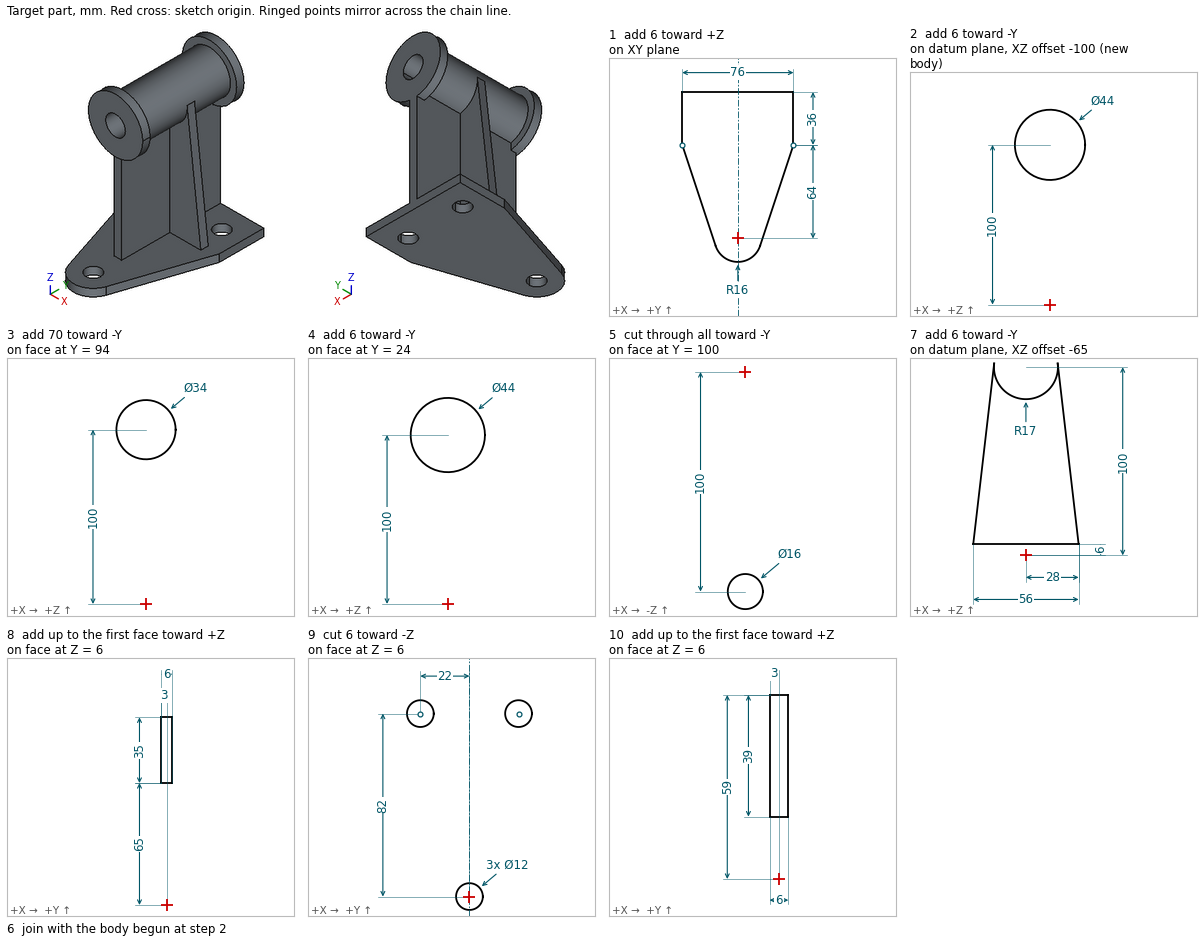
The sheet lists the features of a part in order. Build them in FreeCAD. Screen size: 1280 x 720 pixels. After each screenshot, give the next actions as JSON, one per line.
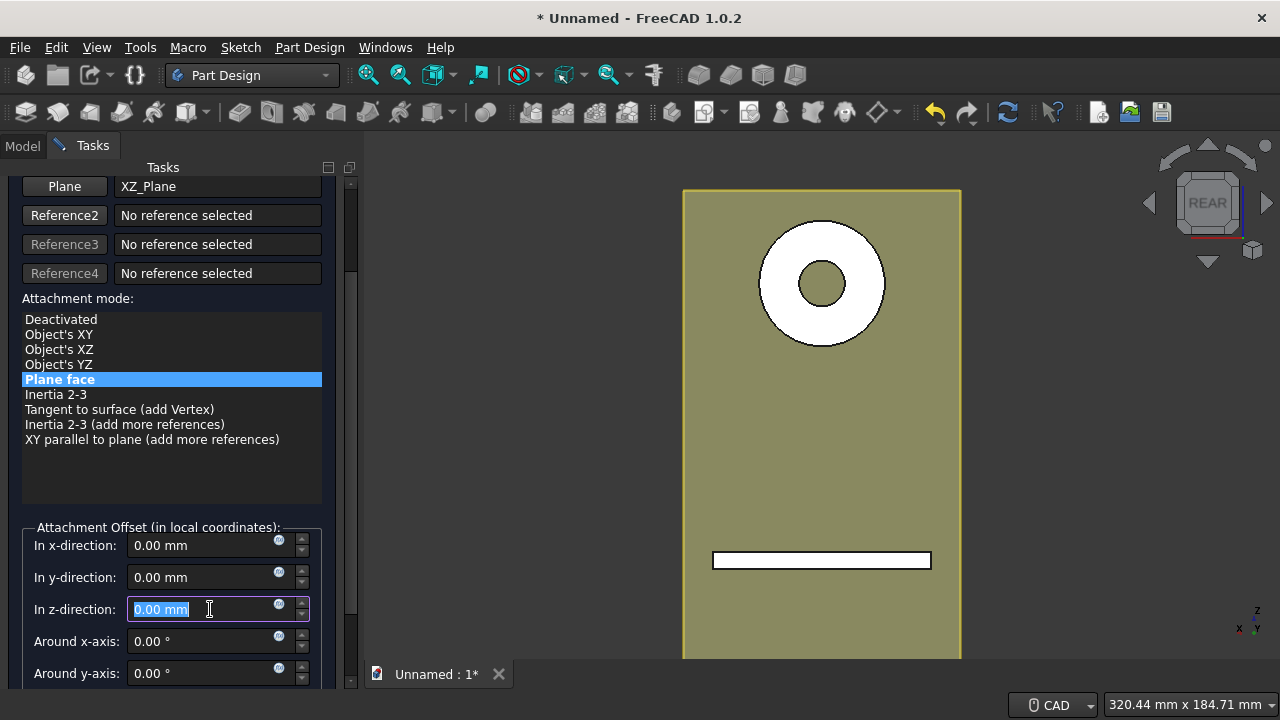
{"action": "type", "text": "-65"}
{"action": "key", "text": "Tab"}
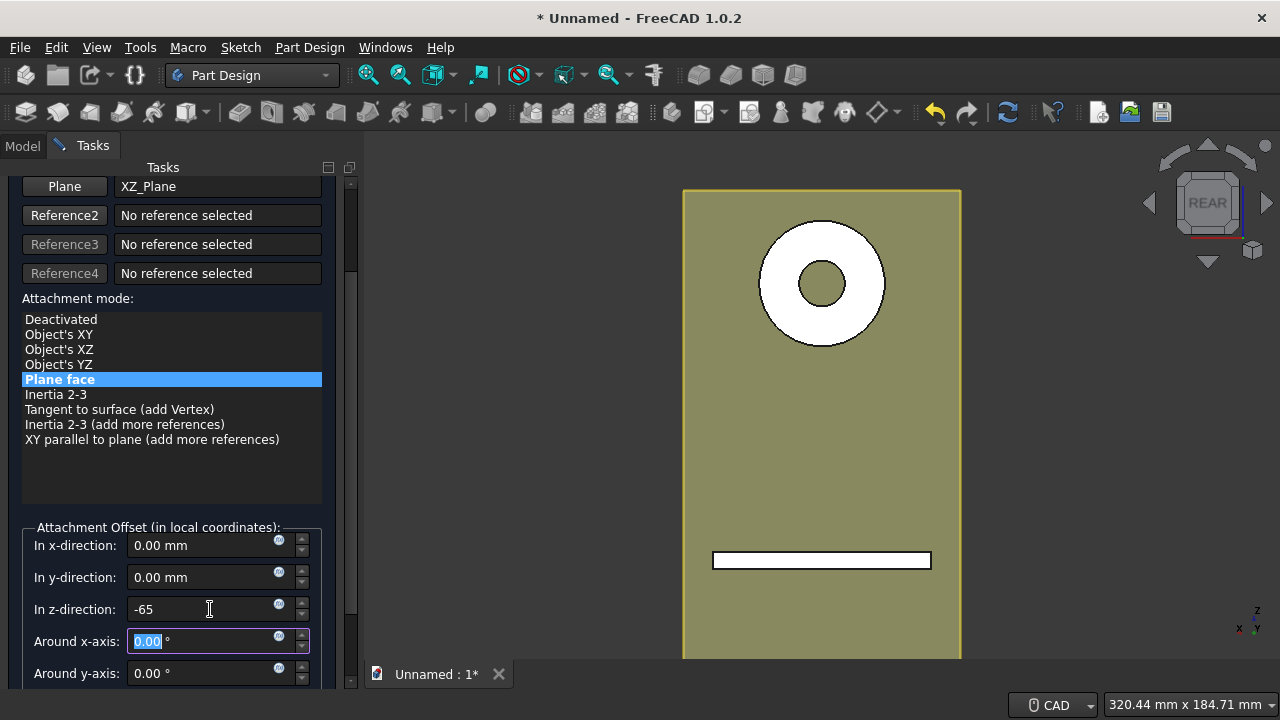
{"action": "scroll", "coordinate": [351, 432], "scroll_direction": "up", "scroll_amount": 3}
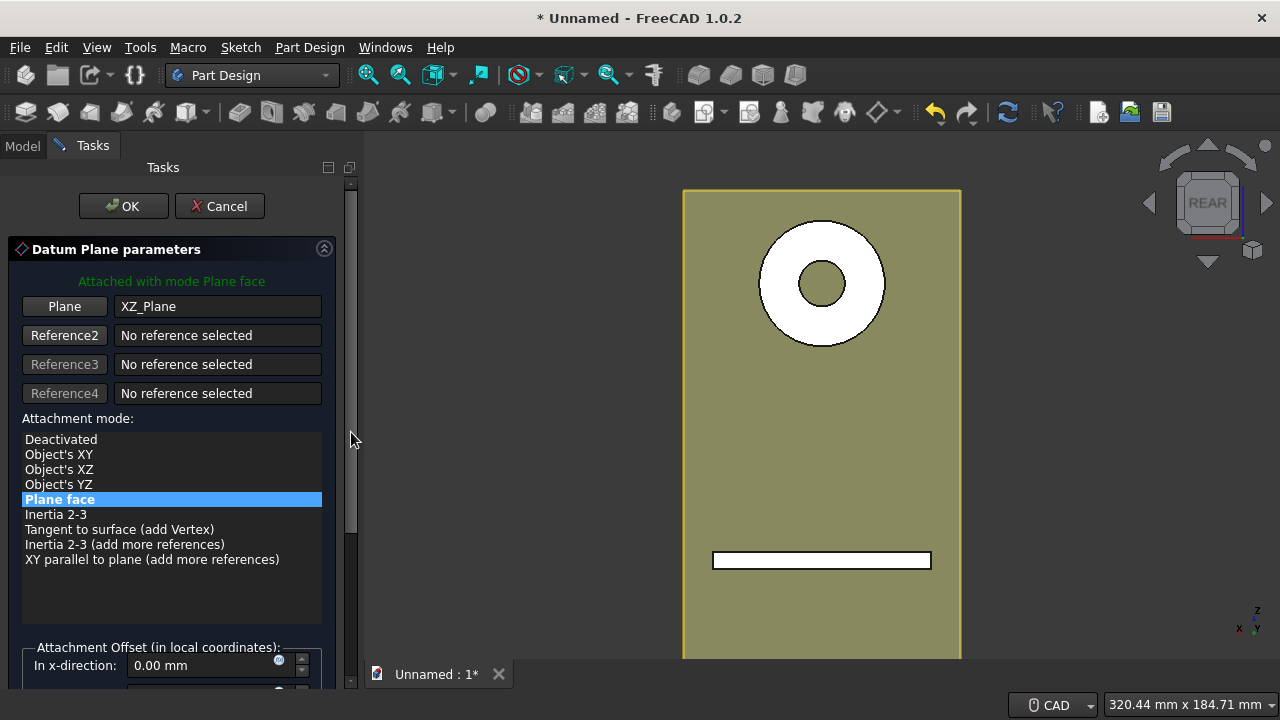
{"action": "left_click", "coordinate": [124, 206]}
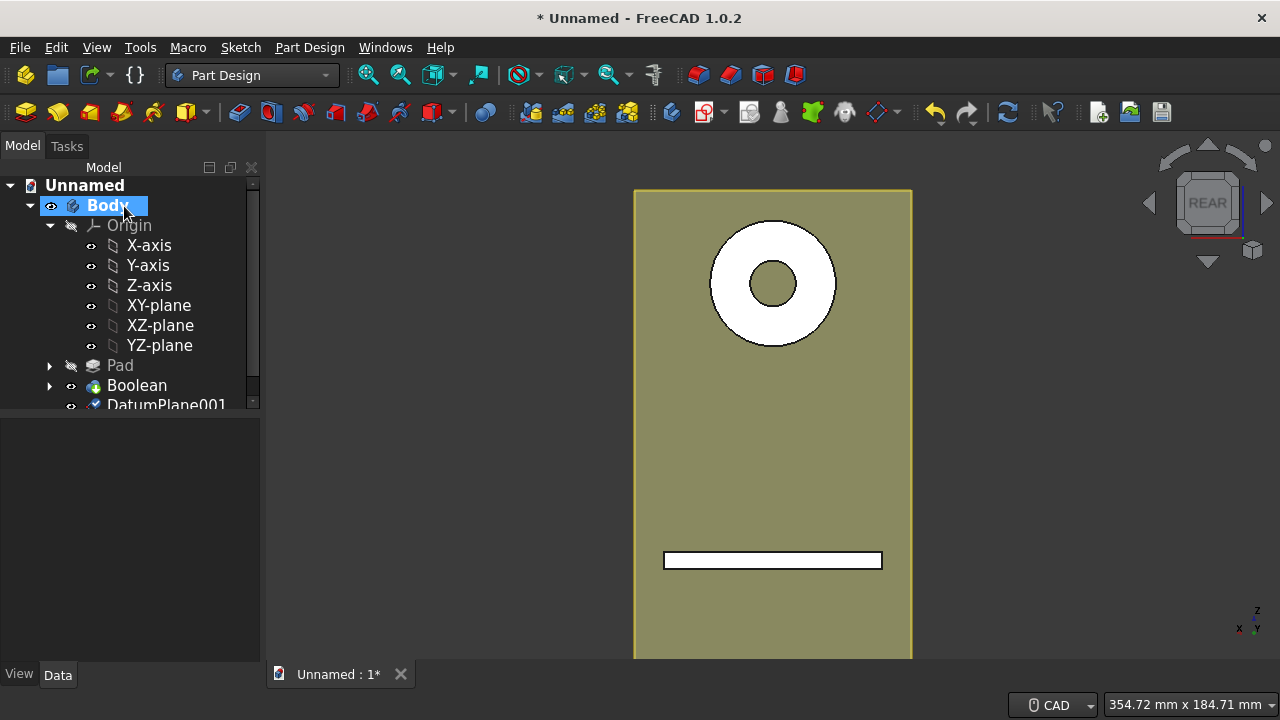
{"action": "left_click", "coordinate": [116, 406]}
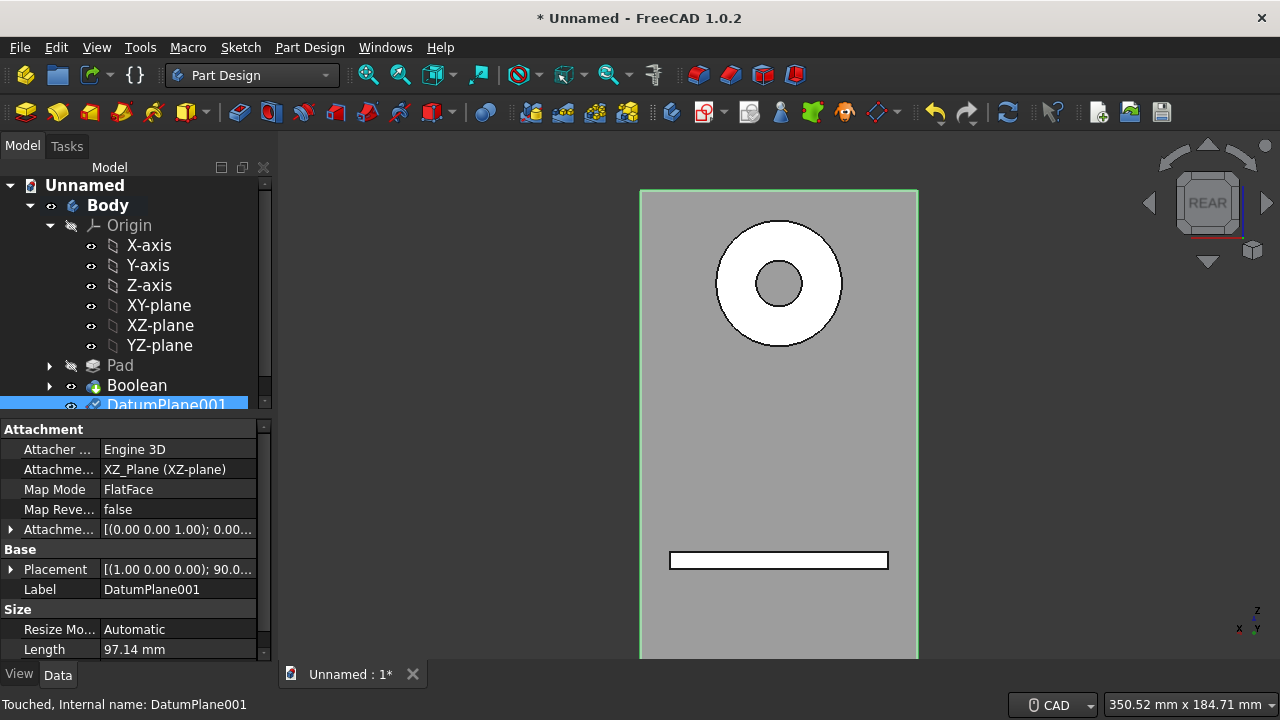
{"action": "left_click", "coordinate": [704, 112]}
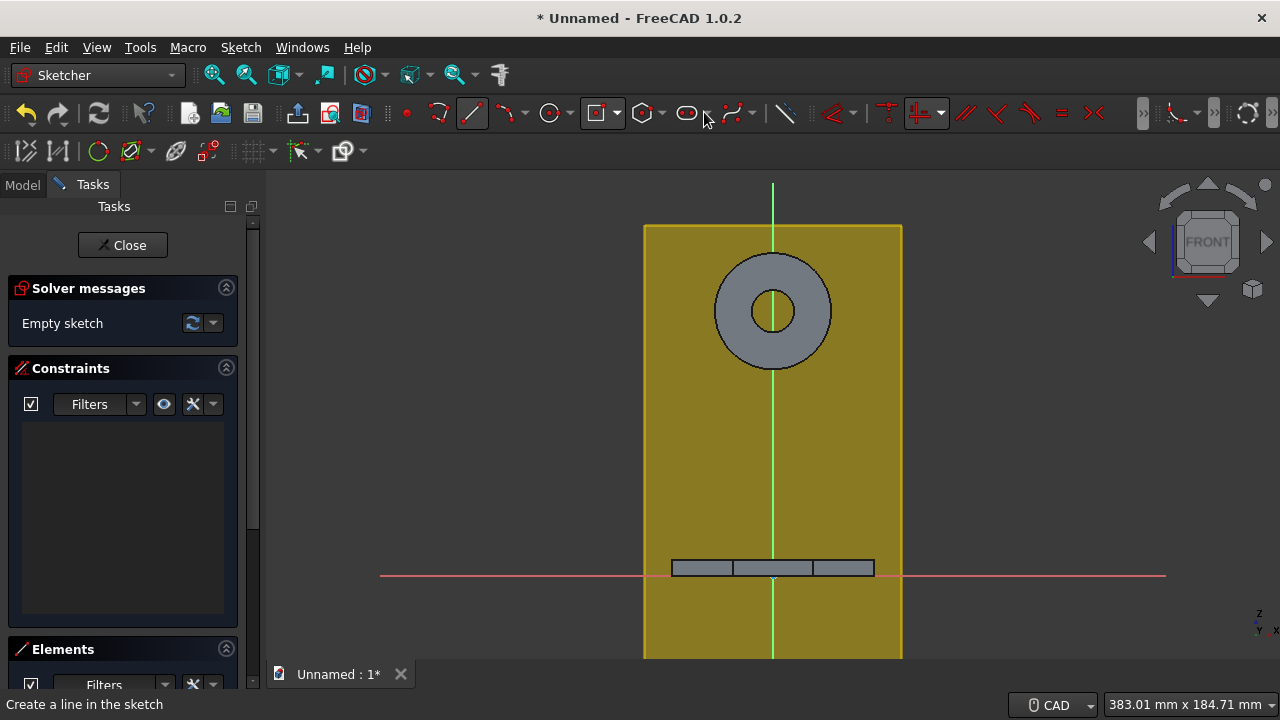
{"action": "key", "text": "q s"}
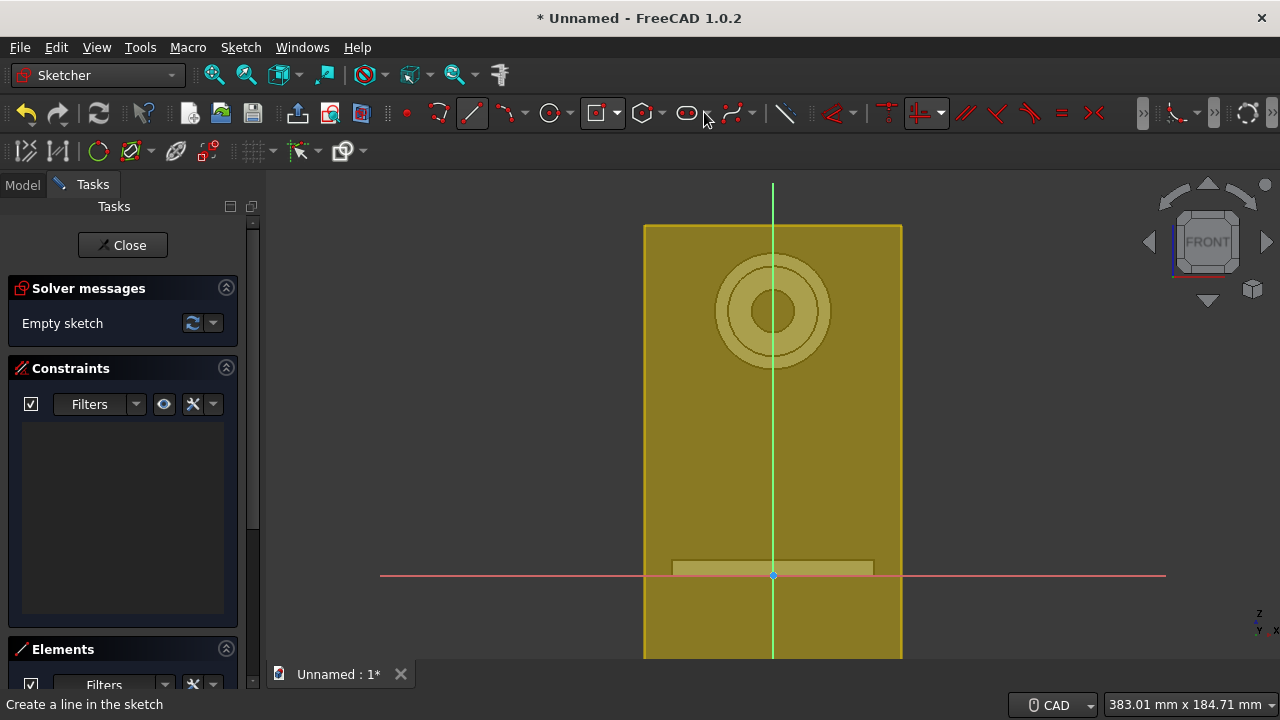
{"action": "key", "text": "g m"}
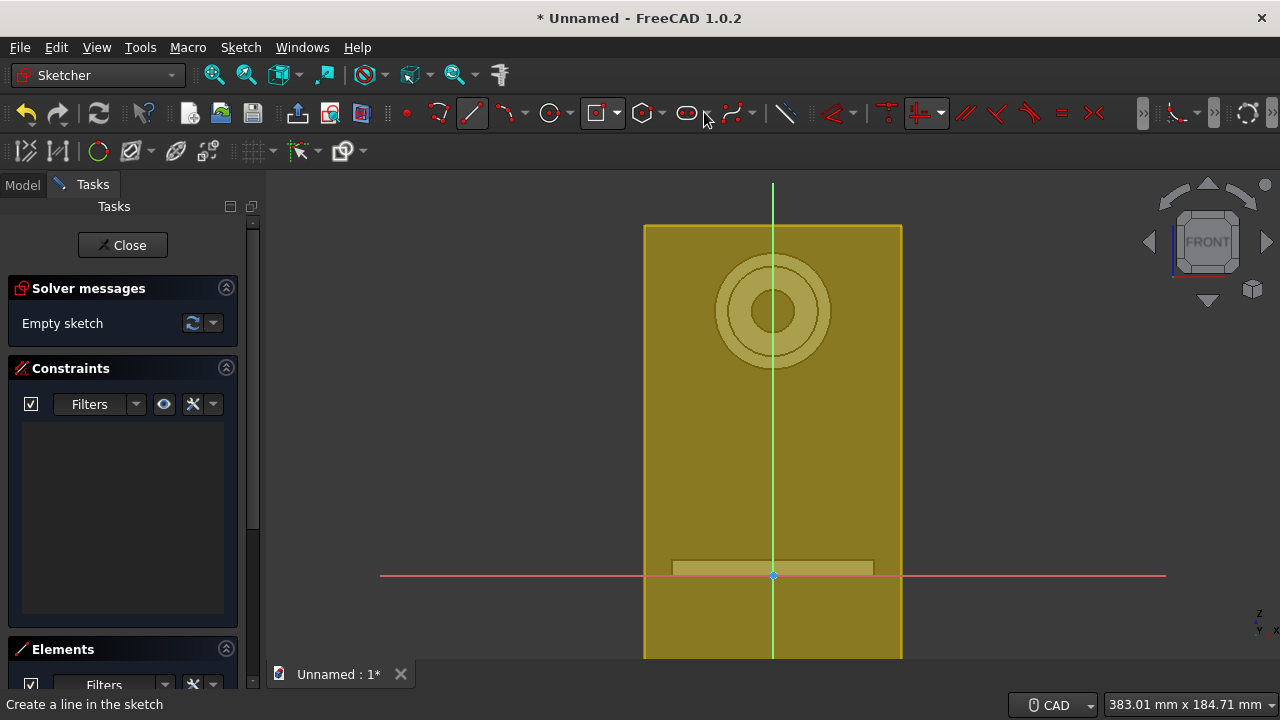
{"action": "left_click", "coordinate": [818, 306]}
{"action": "left_click", "coordinate": [847, 560]}
{"action": "left_click", "coordinate": [699, 560]}
{"action": "left_click", "coordinate": [728, 306]}
{"action": "right_click", "coordinate": [728, 306]}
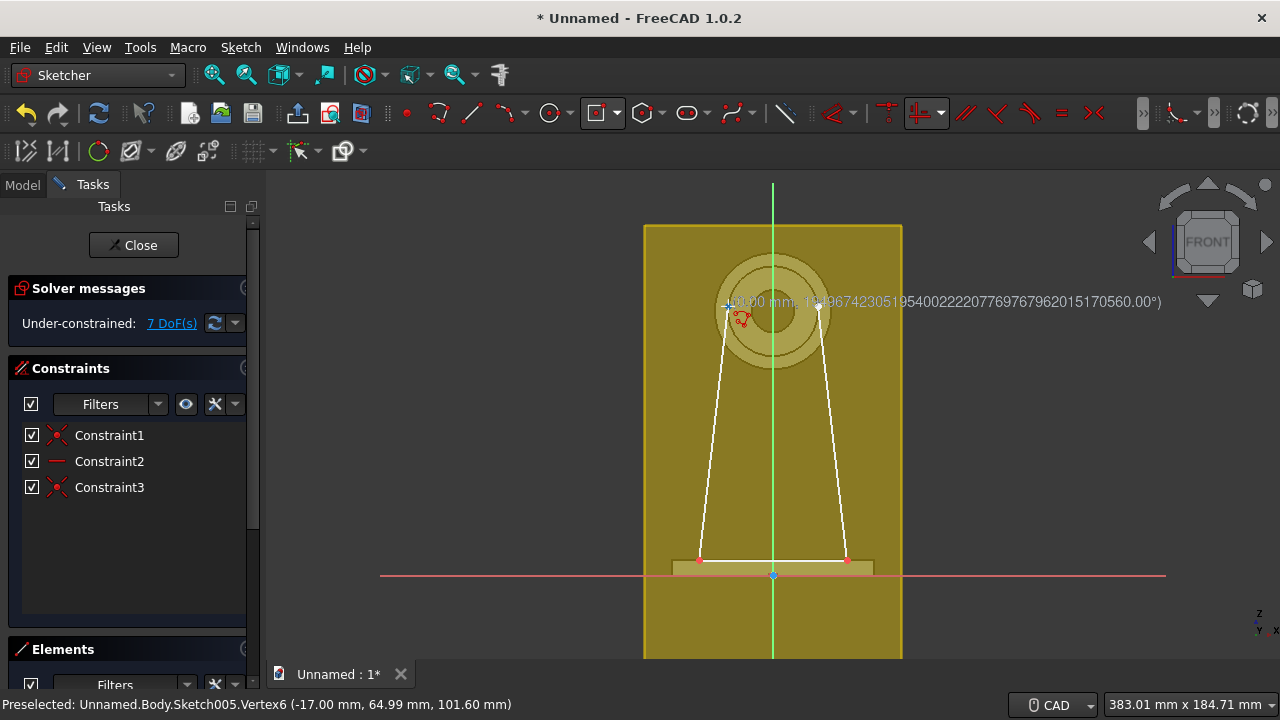
{"action": "left_click", "coordinate": [506, 114]}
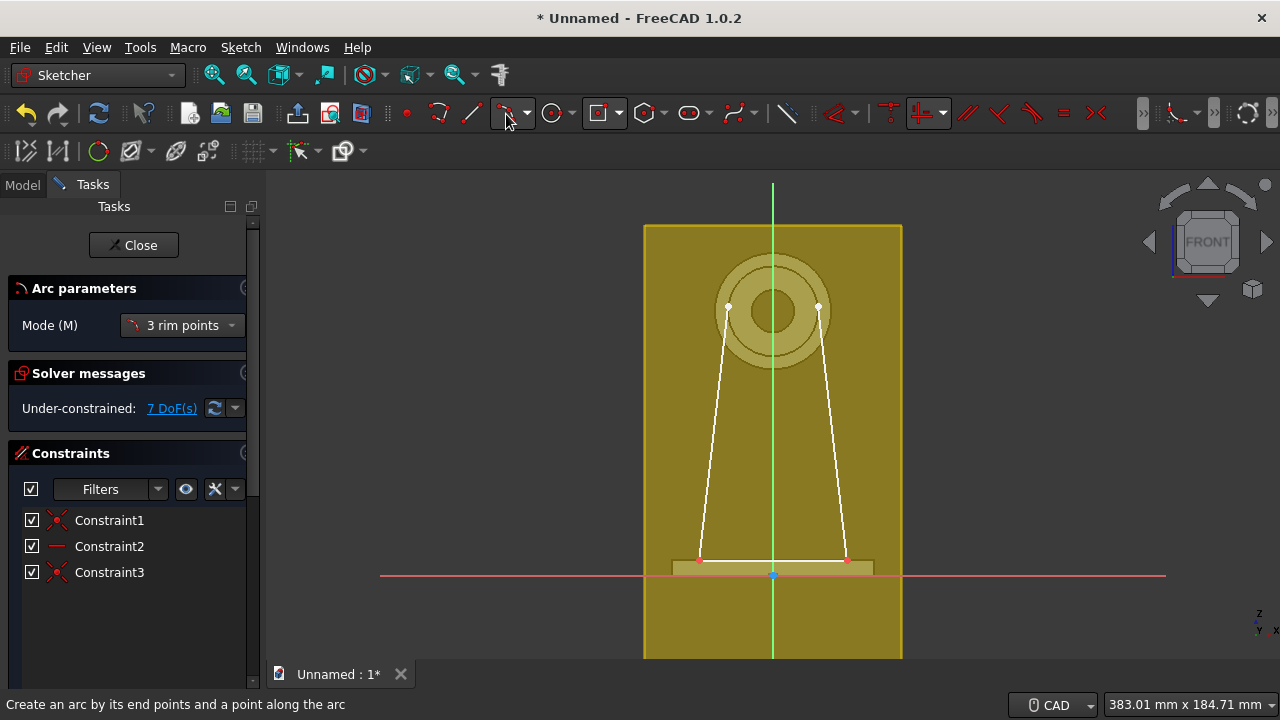
{"action": "left_click", "coordinate": [728, 307]}
{"action": "left_click", "coordinate": [818, 307]}
{"action": "left_click", "coordinate": [758, 354]}
{"action": "key", "text": "Escape"}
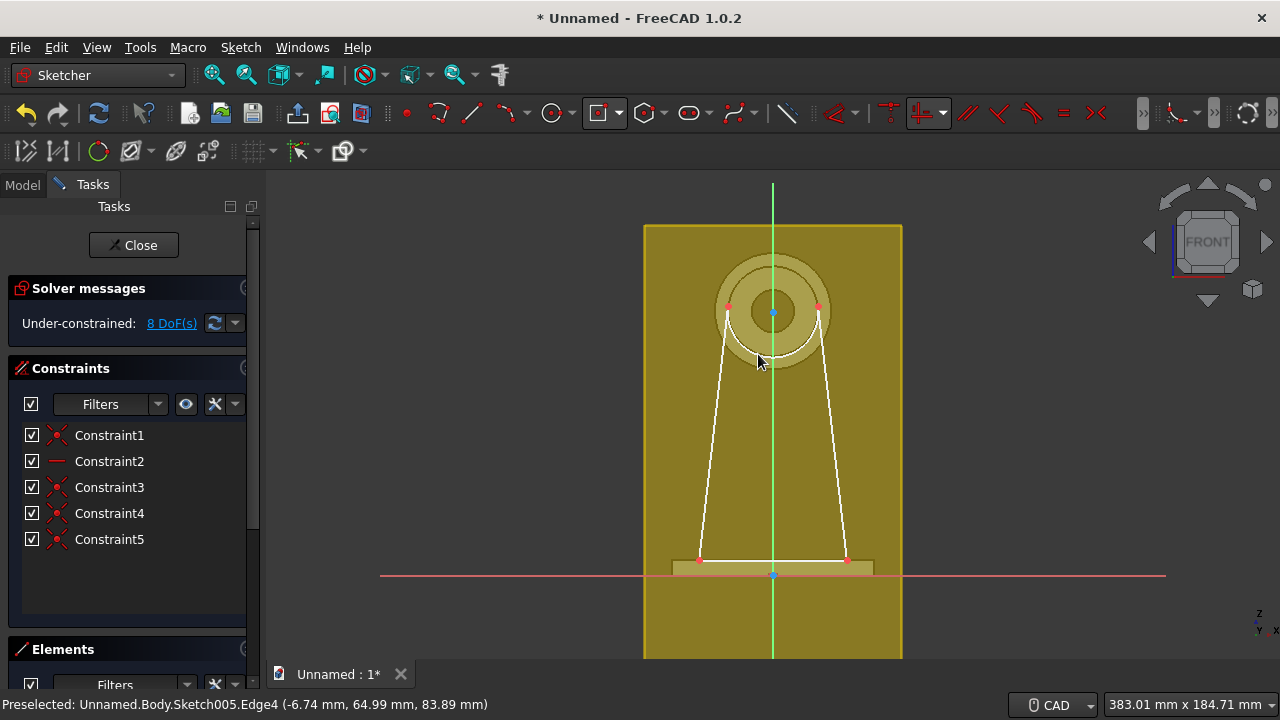
{"action": "left_click", "coordinate": [827, 383]}